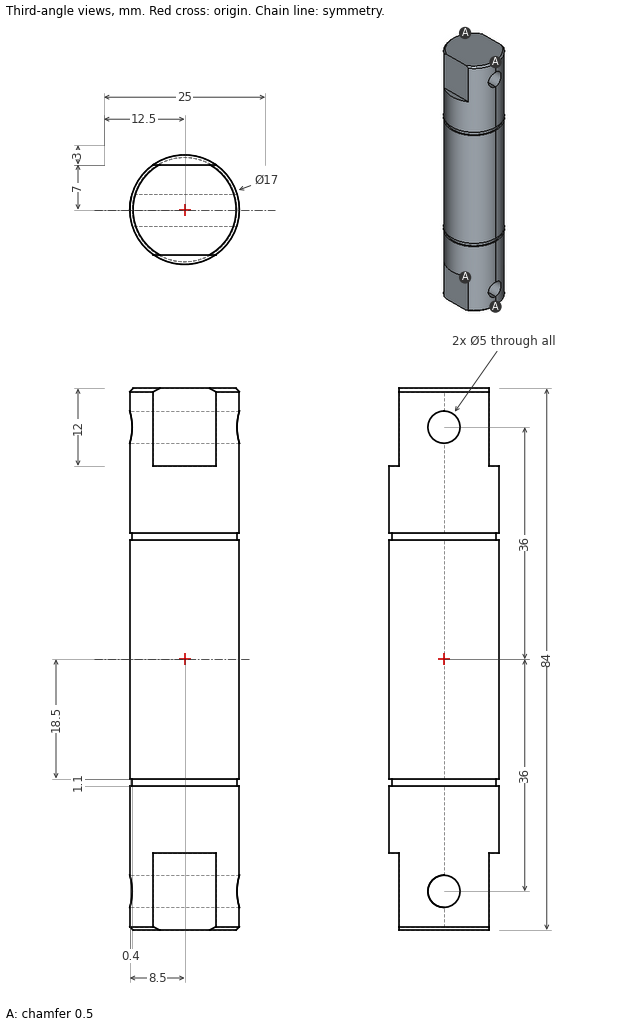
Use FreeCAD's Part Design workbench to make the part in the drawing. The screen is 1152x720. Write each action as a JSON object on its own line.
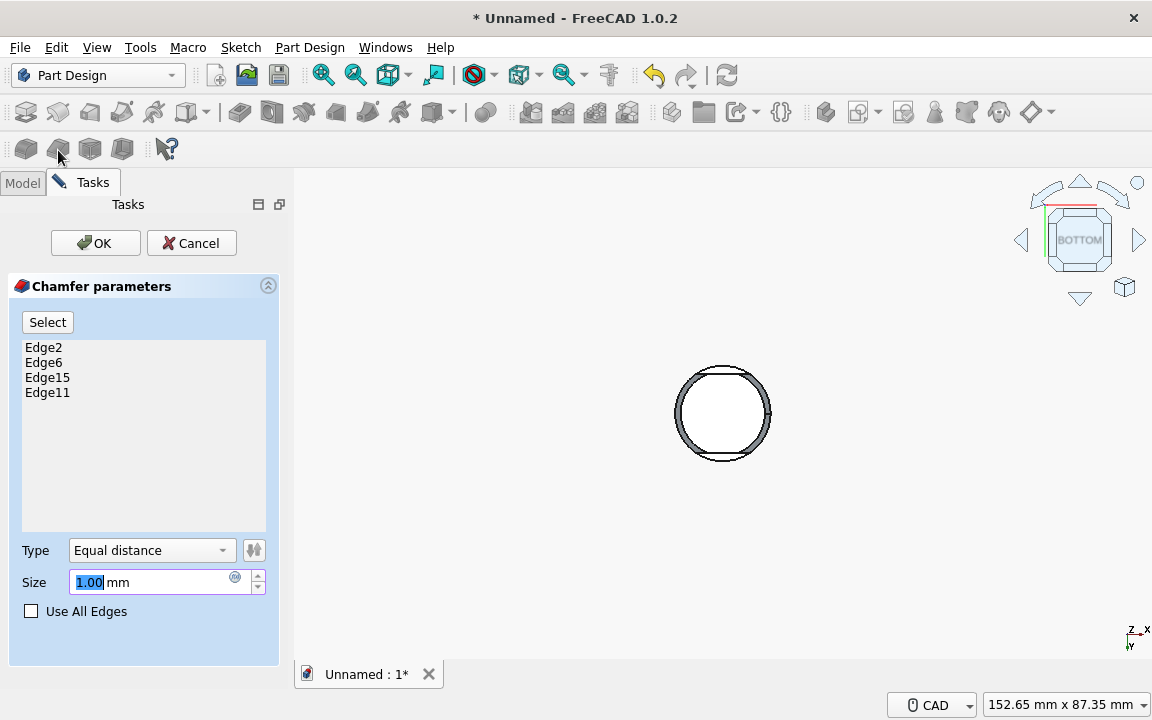
{"action": "type", "text": "0.5"}
{"action": "key", "text": "Tab"}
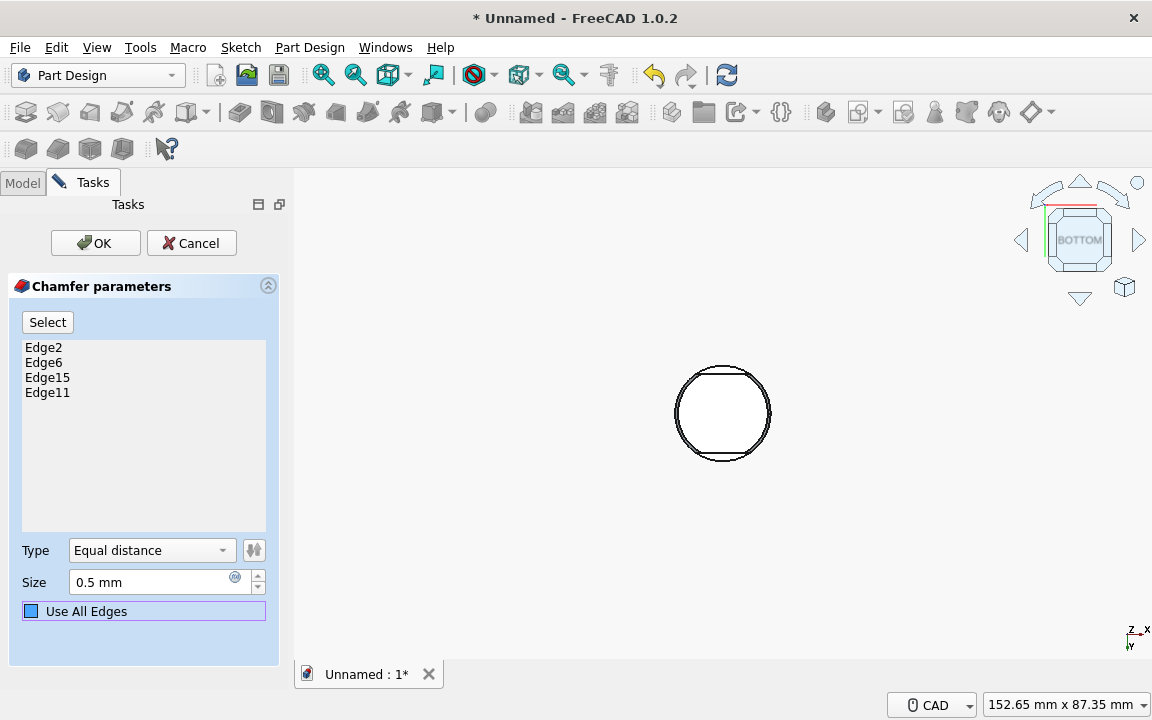
{"action": "left_click", "coordinate": [96, 243]}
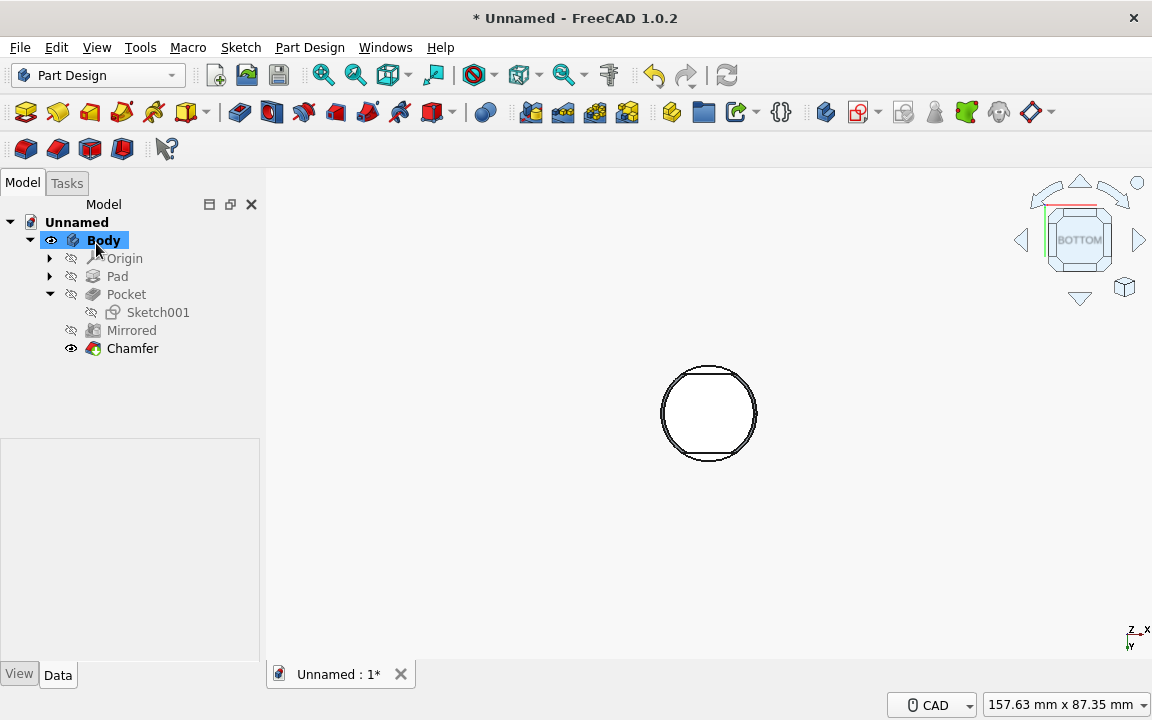
{"action": "left_click", "coordinate": [324, 76]}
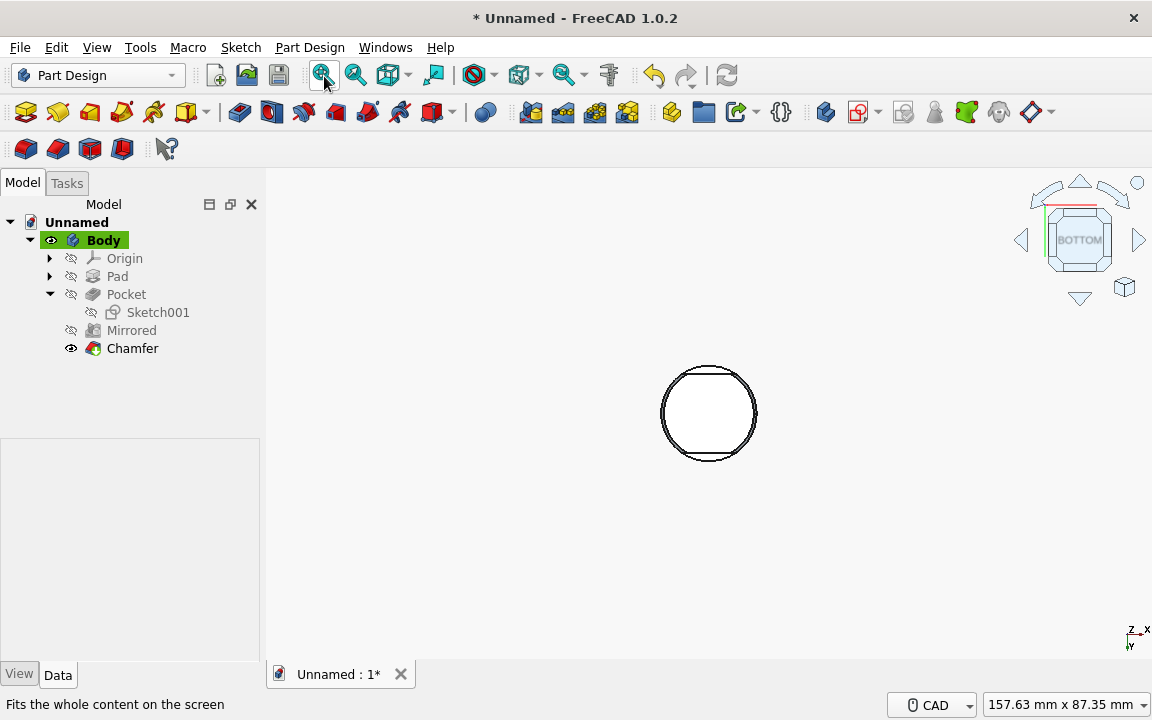
{"action": "left_click", "coordinate": [50, 258]}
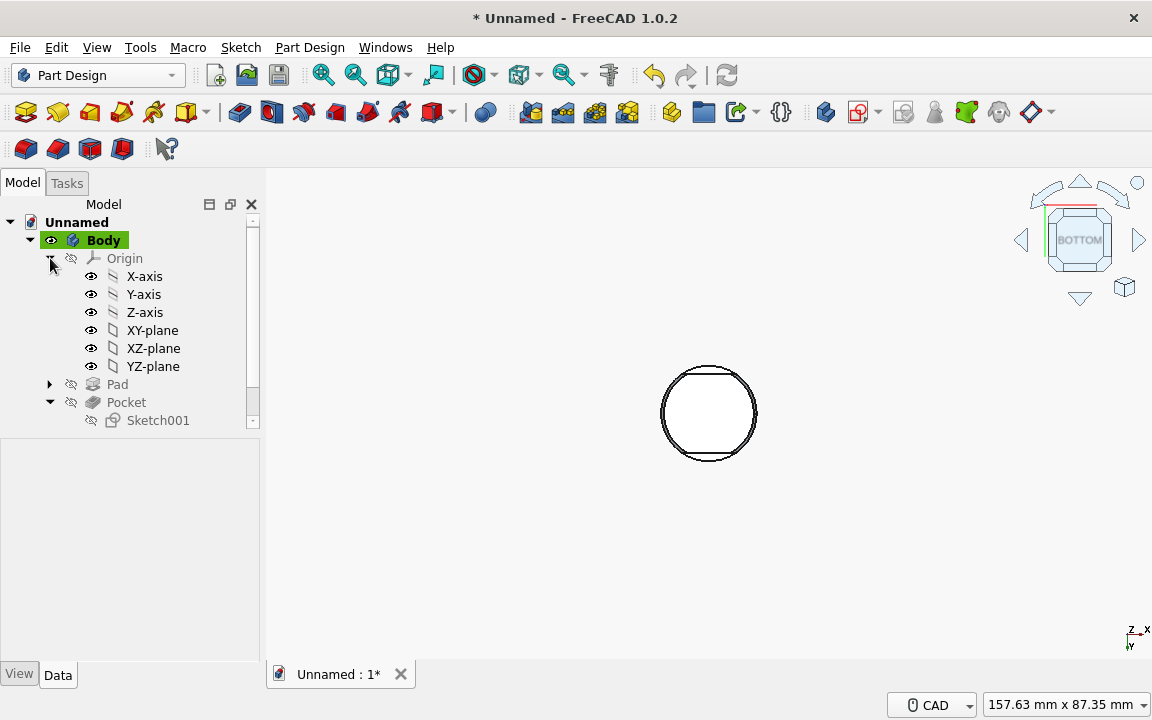
{"action": "left_click", "coordinate": [136, 366]}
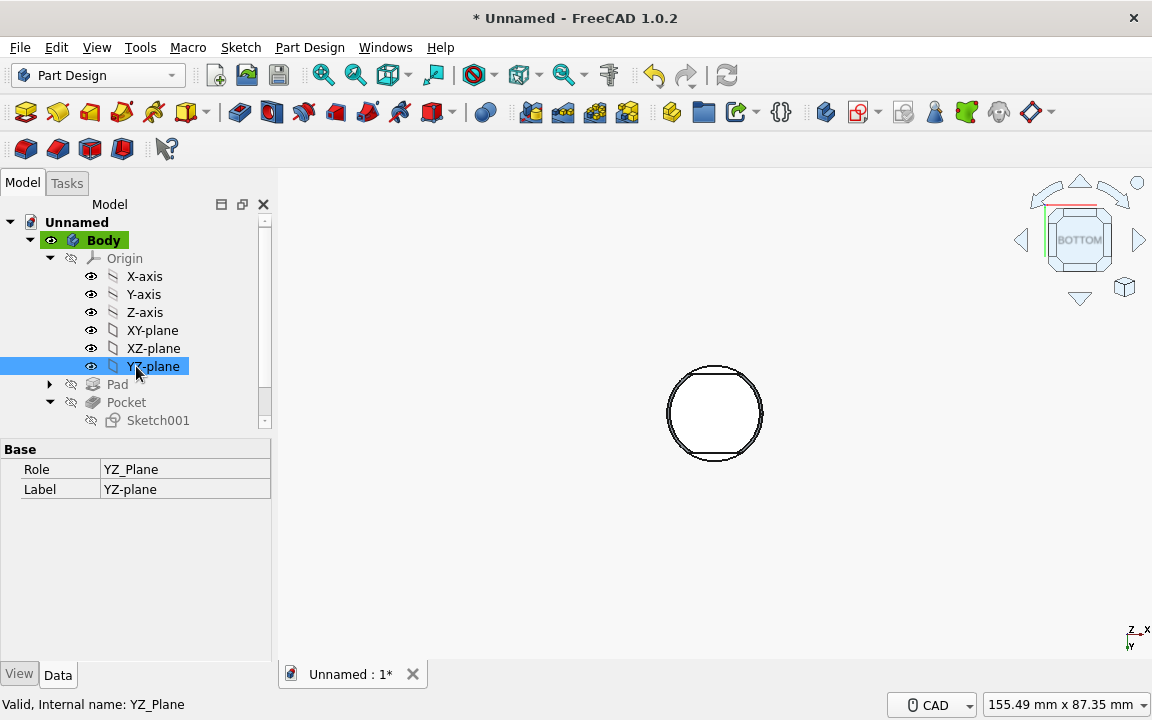
{"action": "left_click", "coordinate": [1032, 112]}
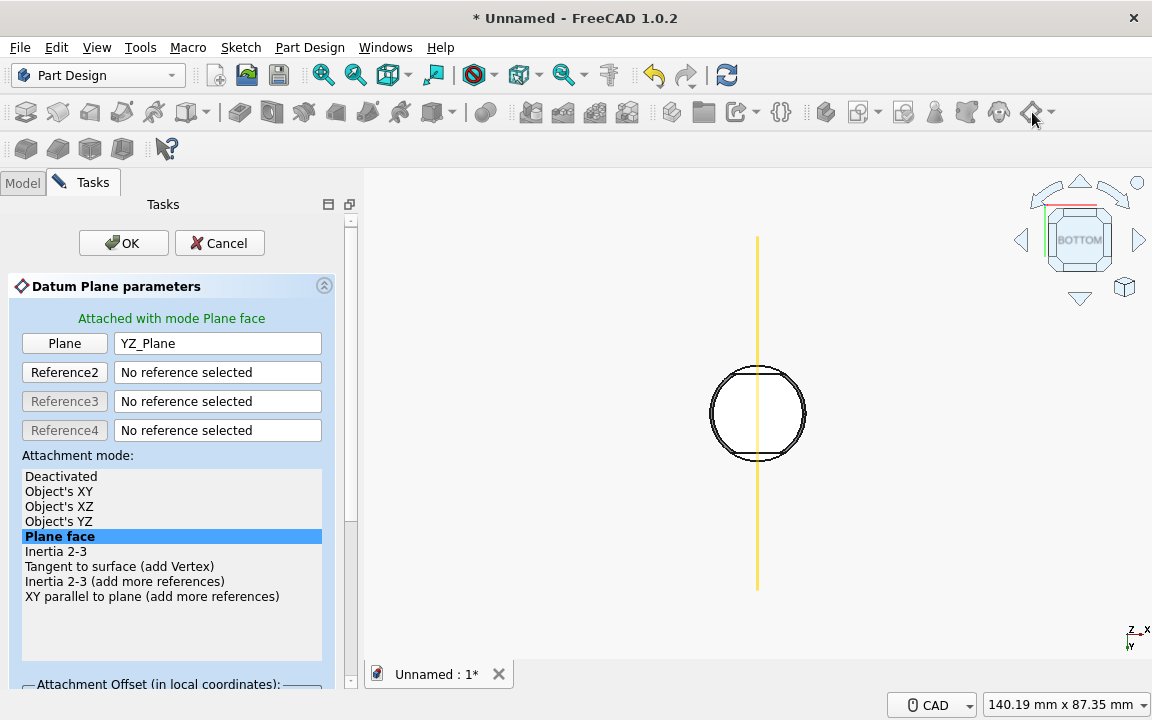
{"action": "scroll", "coordinate": [351, 451], "scroll_direction": "down", "scroll_amount": 3}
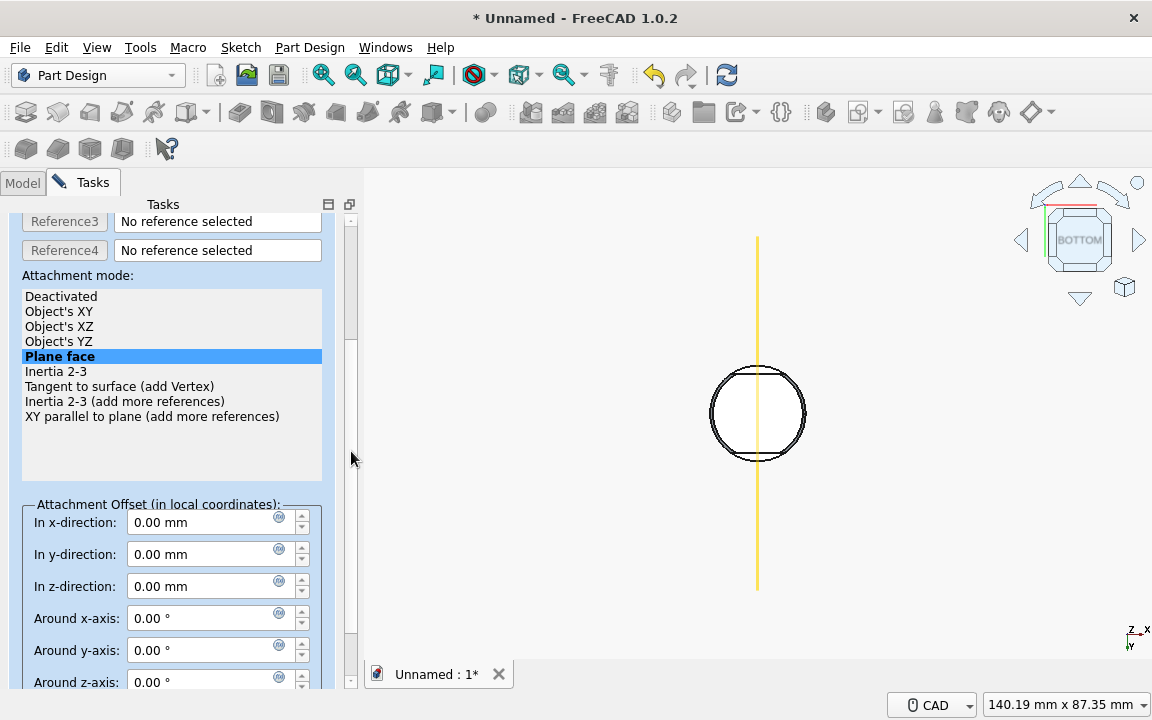
{"action": "triple_click", "coordinate": [210, 586]}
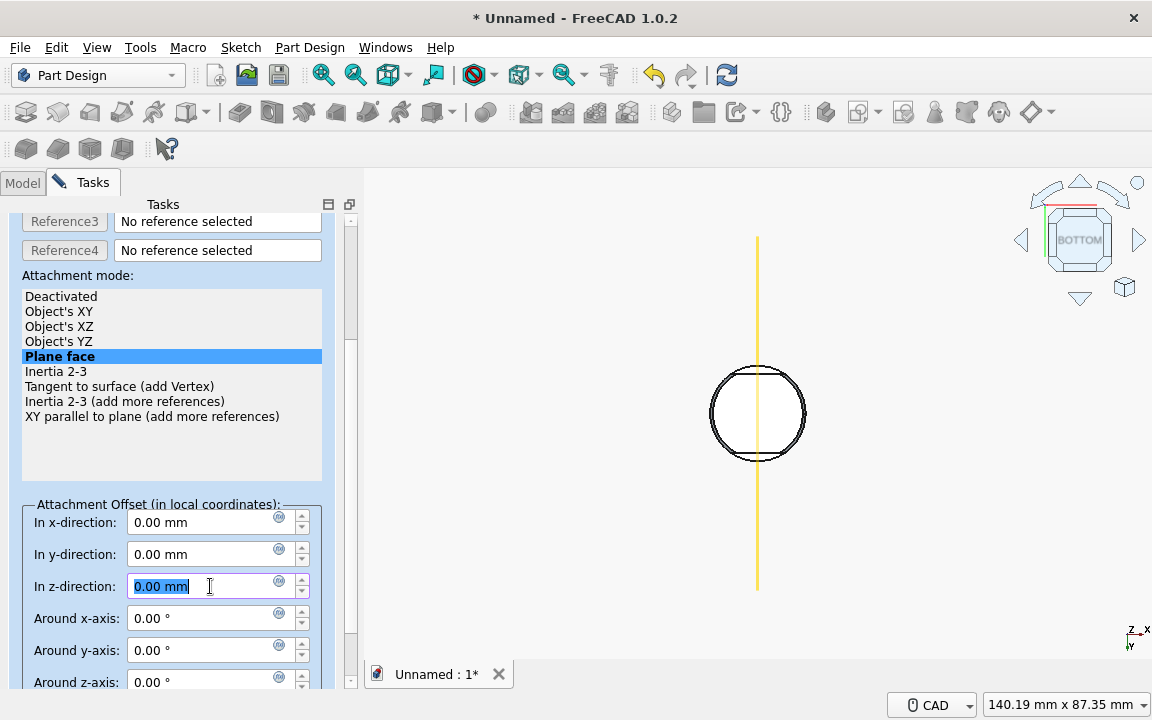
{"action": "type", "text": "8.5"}
{"action": "key", "text": "Tab"}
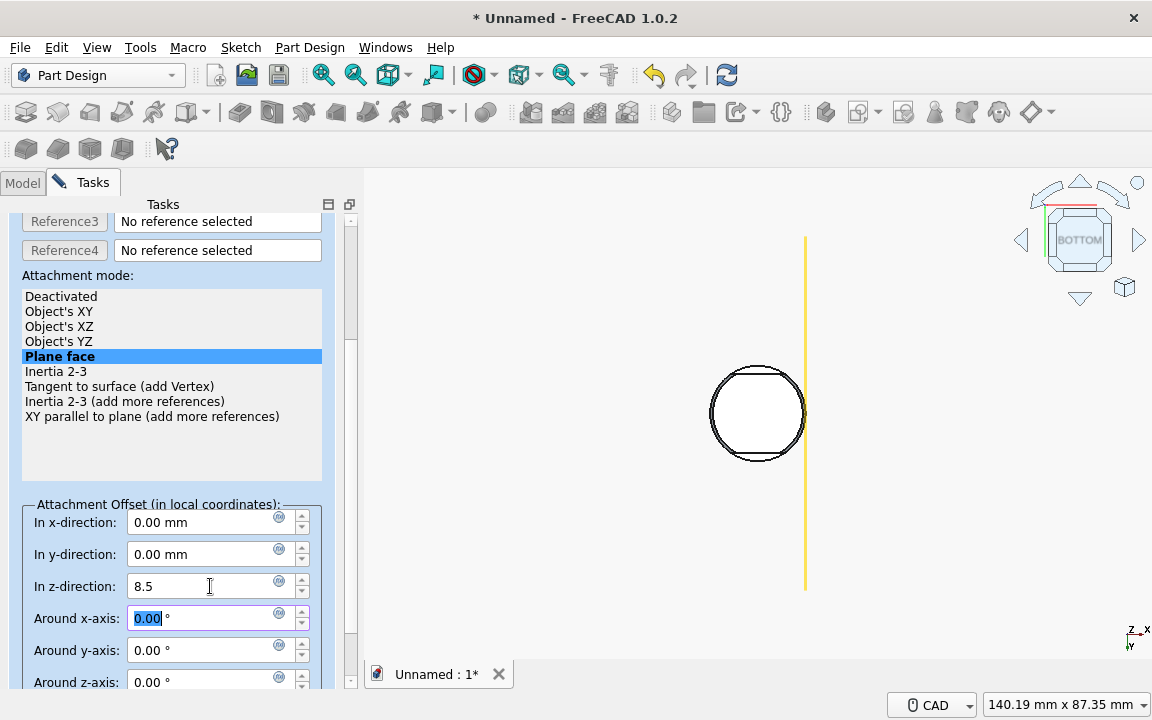
{"action": "scroll", "coordinate": [351, 451], "scroll_direction": "up", "scroll_amount": 4}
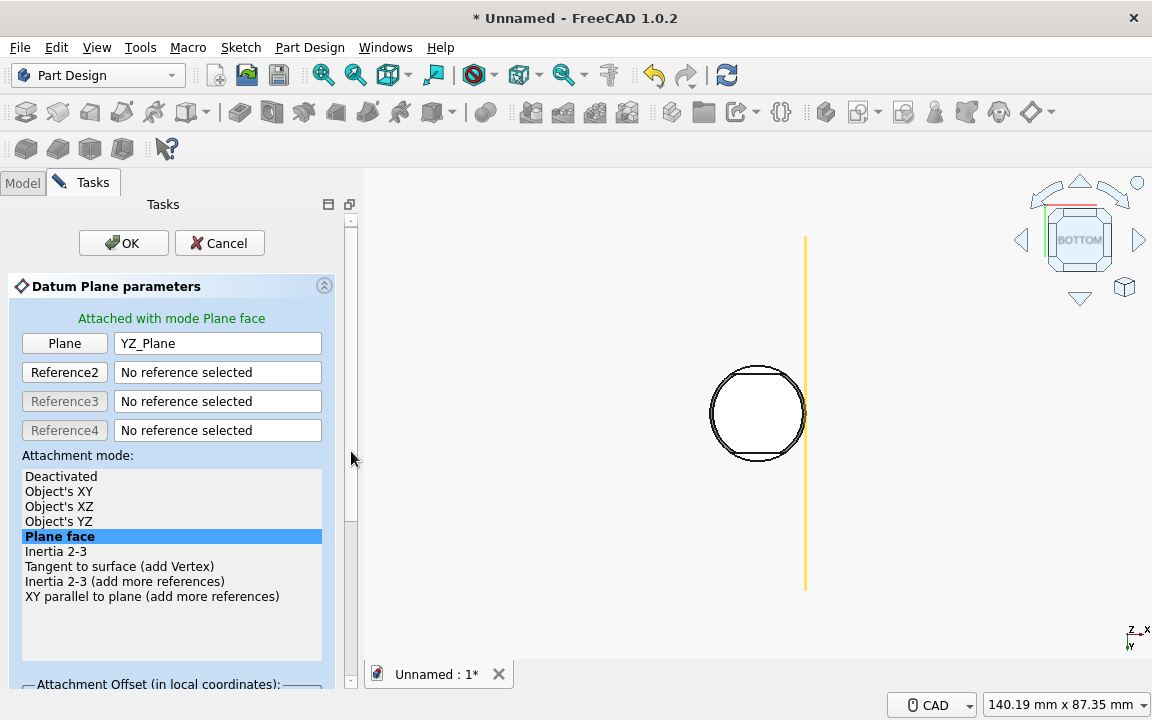
{"action": "left_click", "coordinate": [124, 243]}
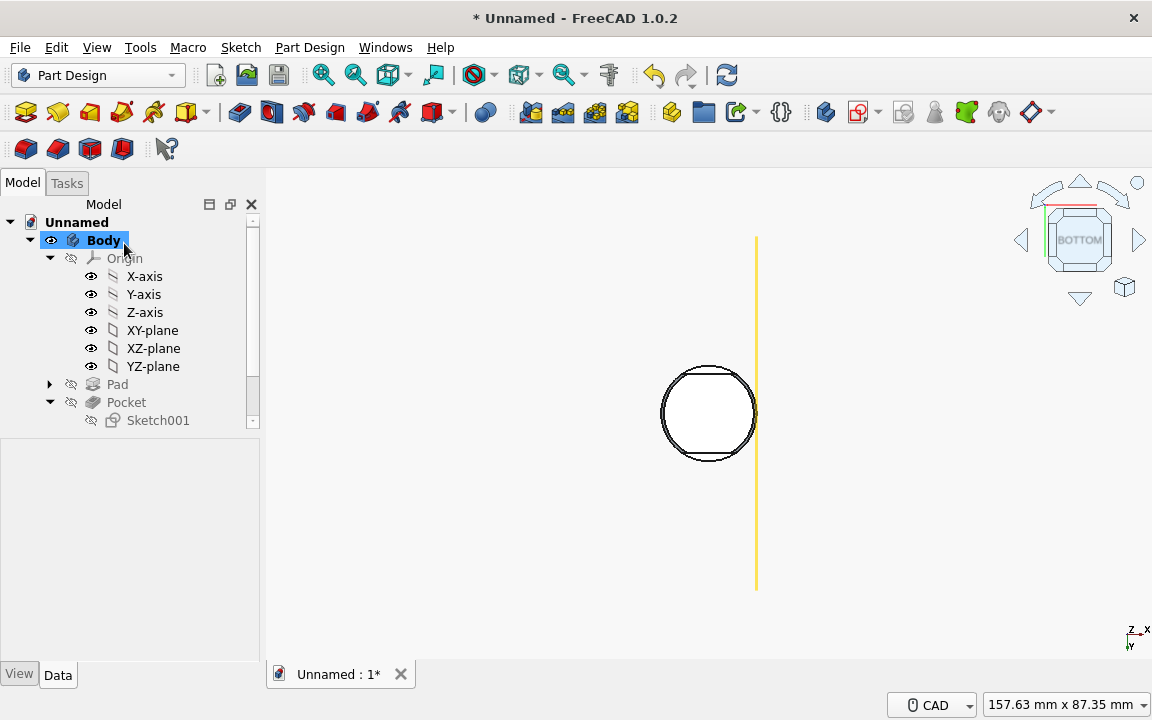
{"action": "scroll", "coordinate": [100, 326], "scroll_direction": "down", "scroll_amount": 3}